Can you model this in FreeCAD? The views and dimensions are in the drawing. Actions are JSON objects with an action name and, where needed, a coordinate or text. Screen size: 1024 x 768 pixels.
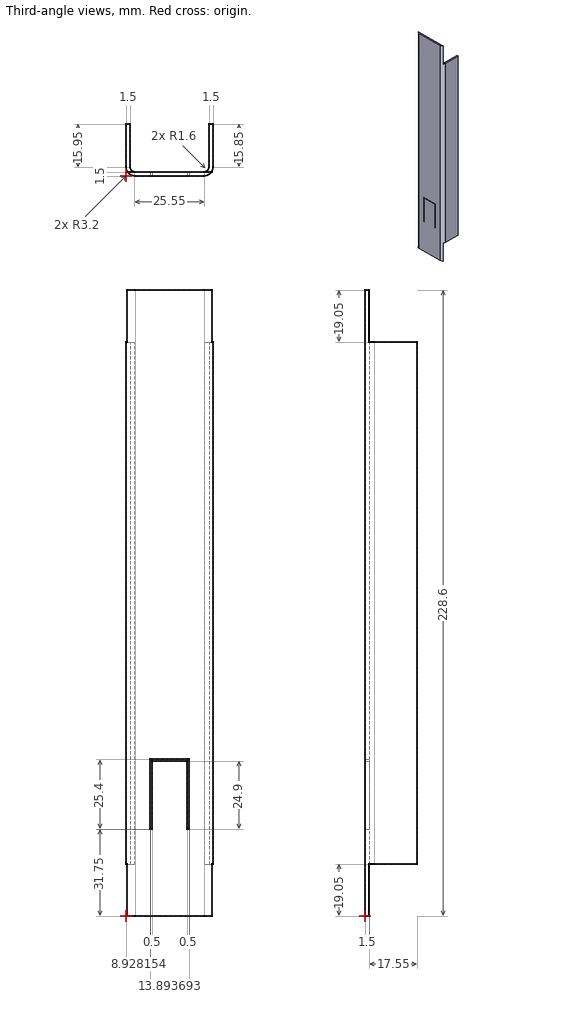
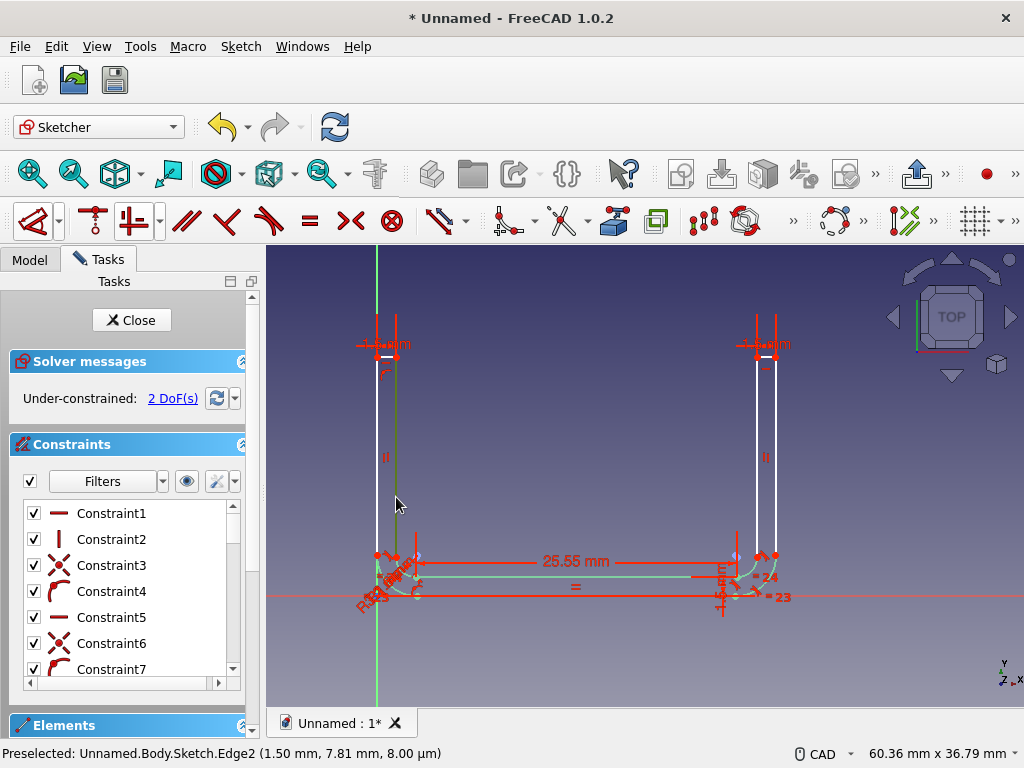
{"action": "left_click", "coordinate": [58, 222]}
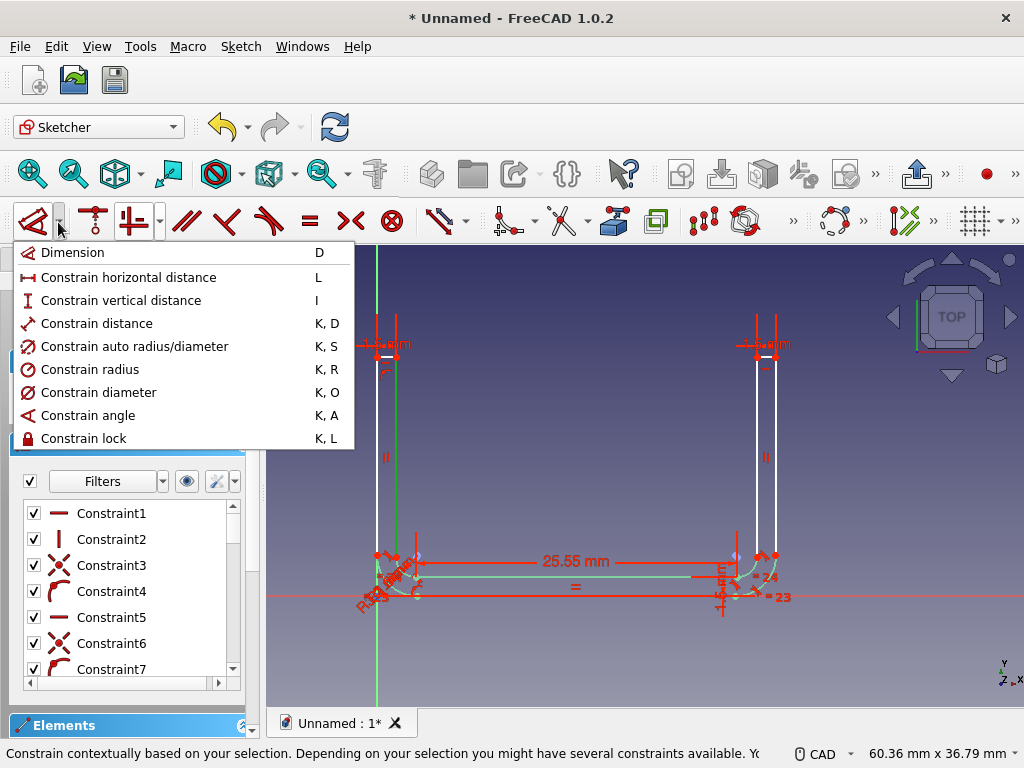
{"action": "left_click", "coordinate": [184, 300]}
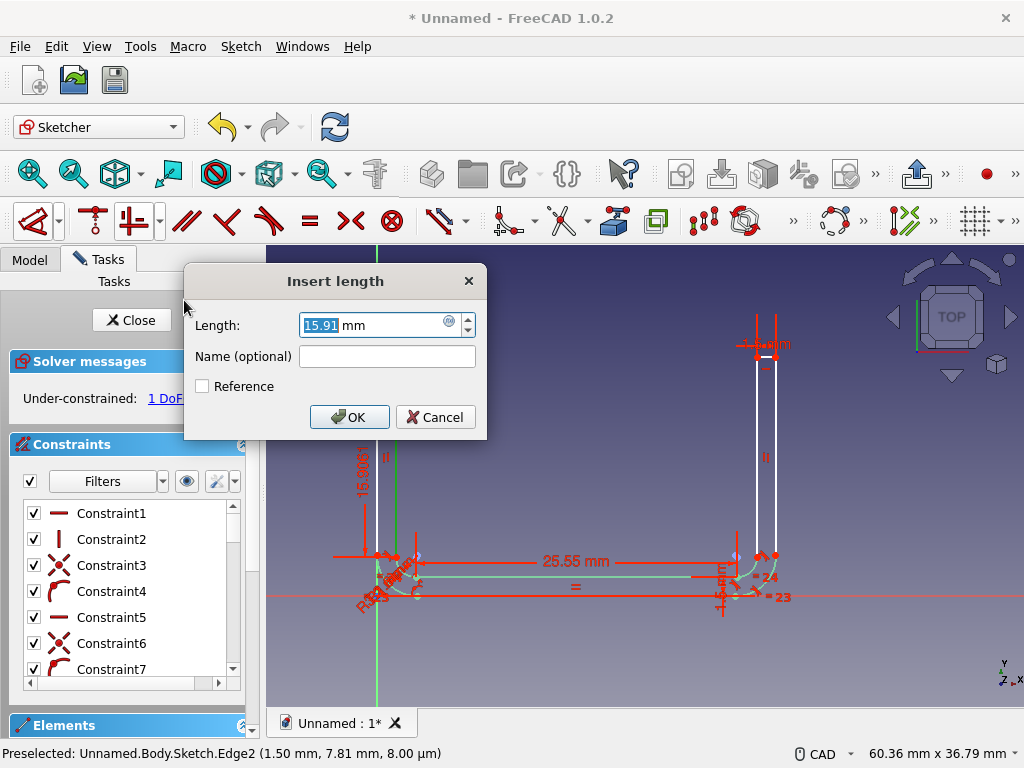
{"action": "type", "text": "15.95"}
{"action": "key", "text": "Return"}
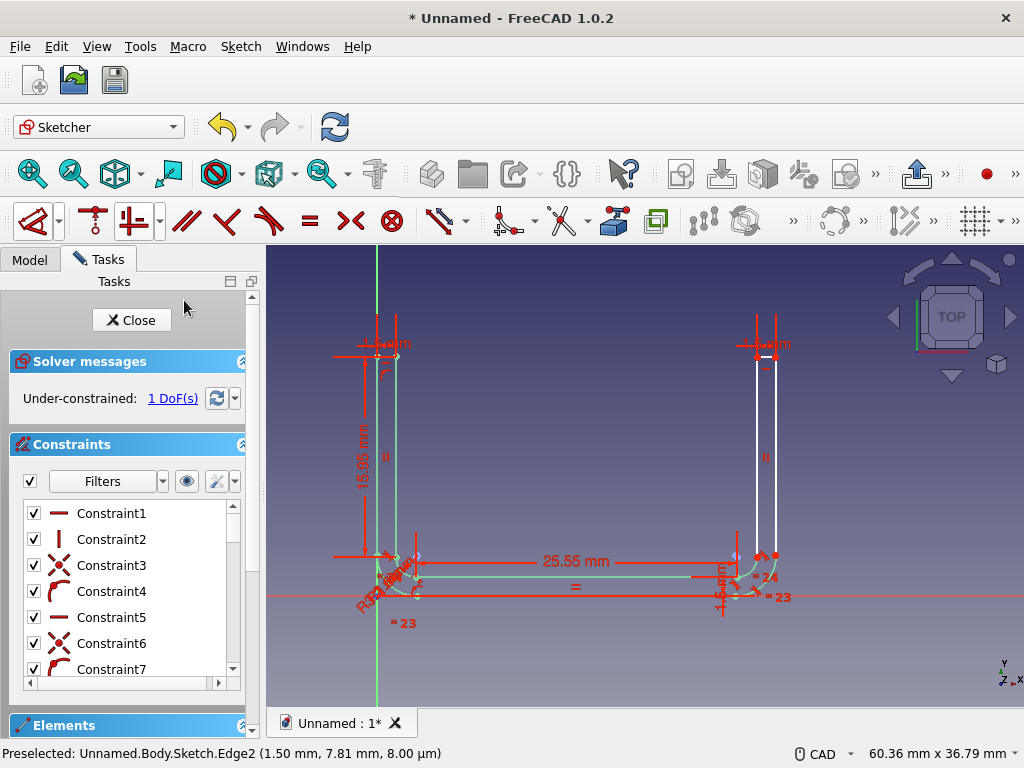
{"action": "left_click", "coordinate": [776, 496]}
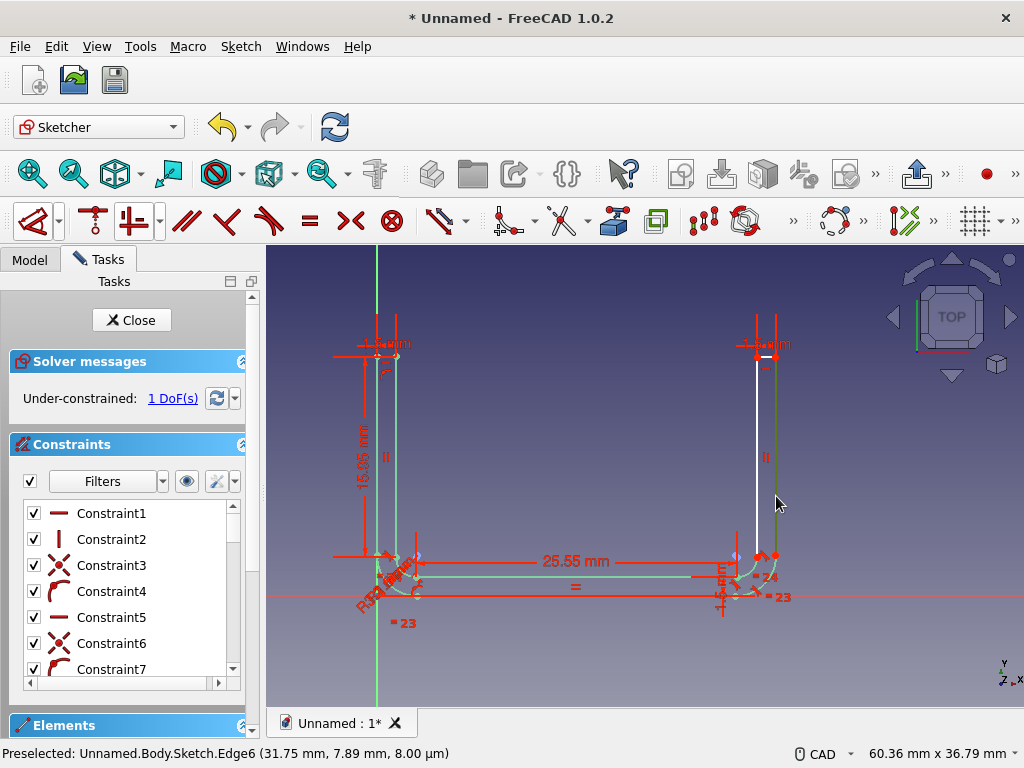
{"action": "left_click", "coordinate": [58, 222]}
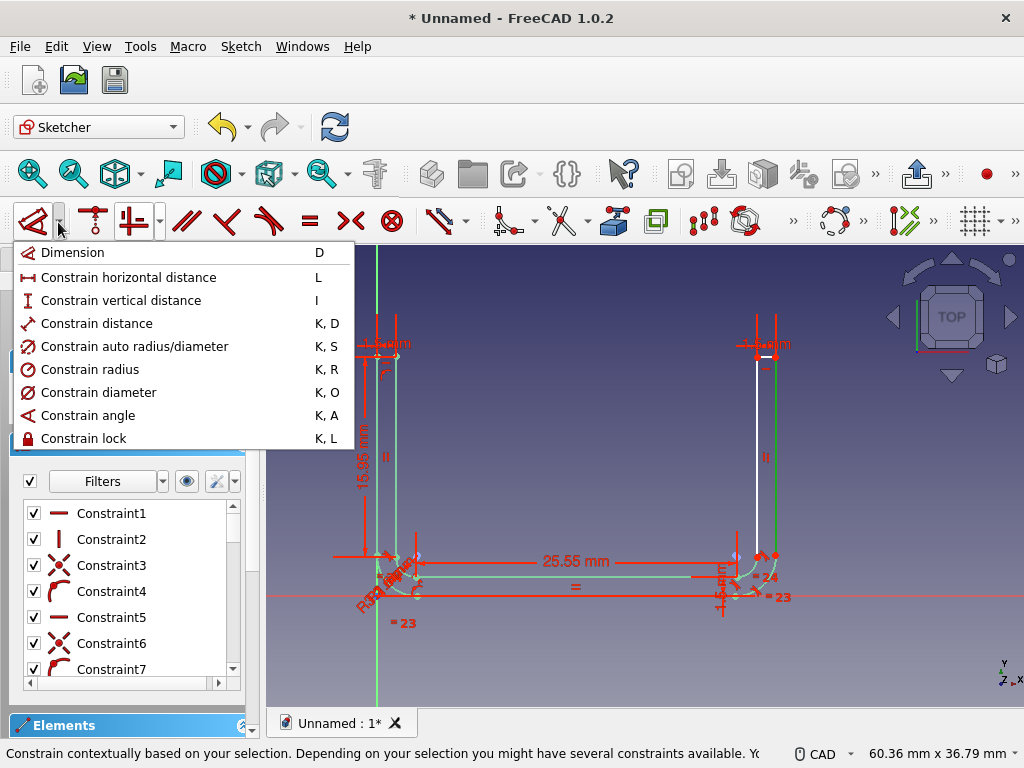
{"action": "left_click", "coordinate": [184, 300]}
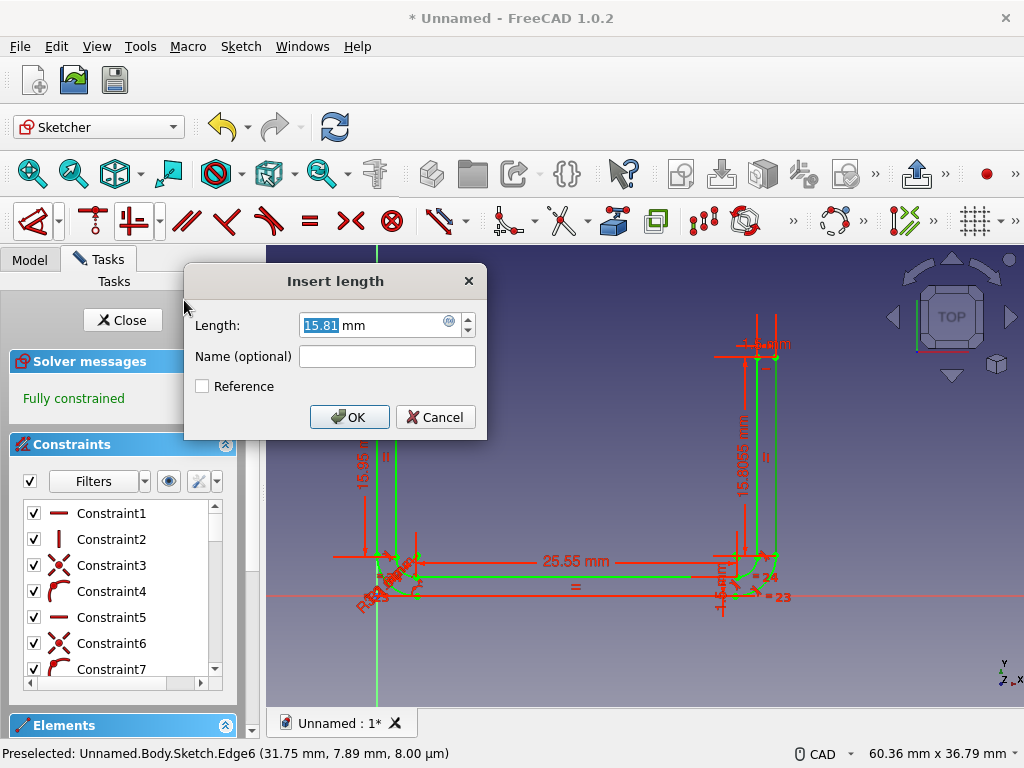
{"action": "type", "text": "15.85"}
{"action": "key", "text": "Return"}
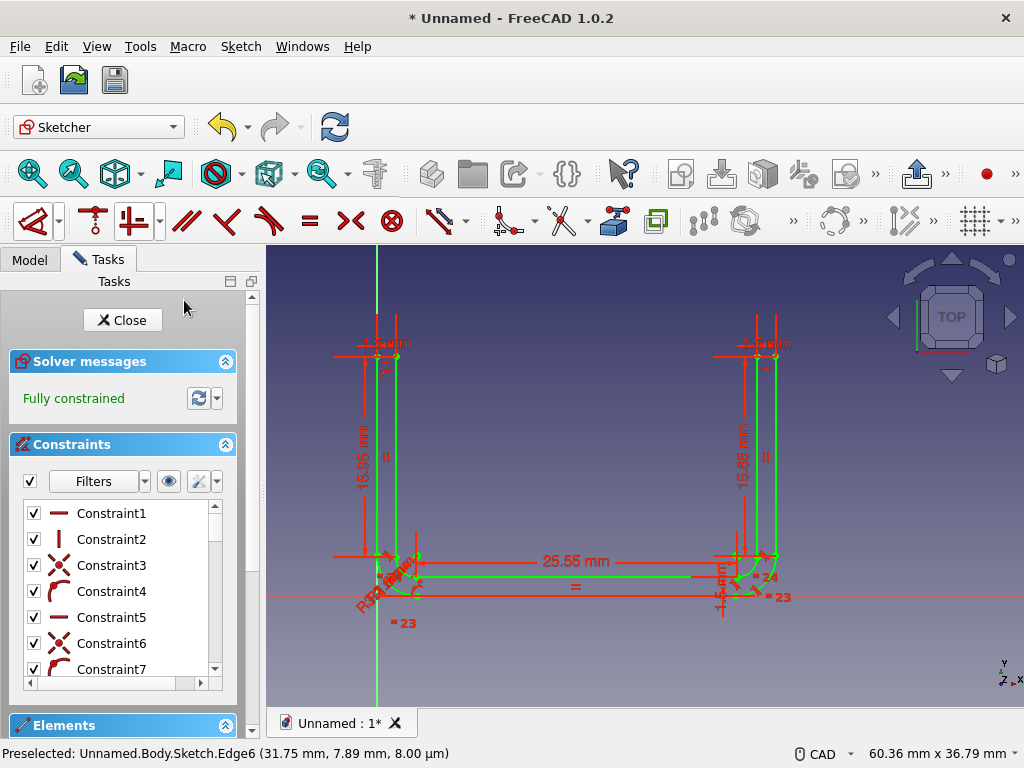
{"action": "left_click", "coordinate": [123, 320]}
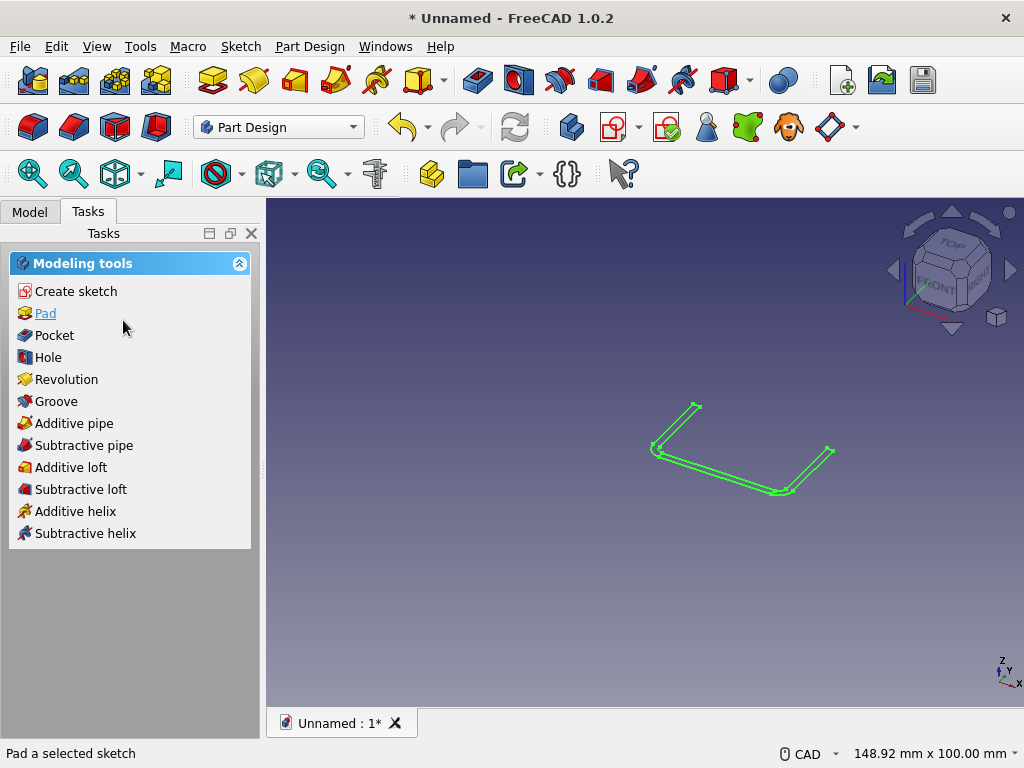
{"action": "left_click", "coordinate": [213, 80]}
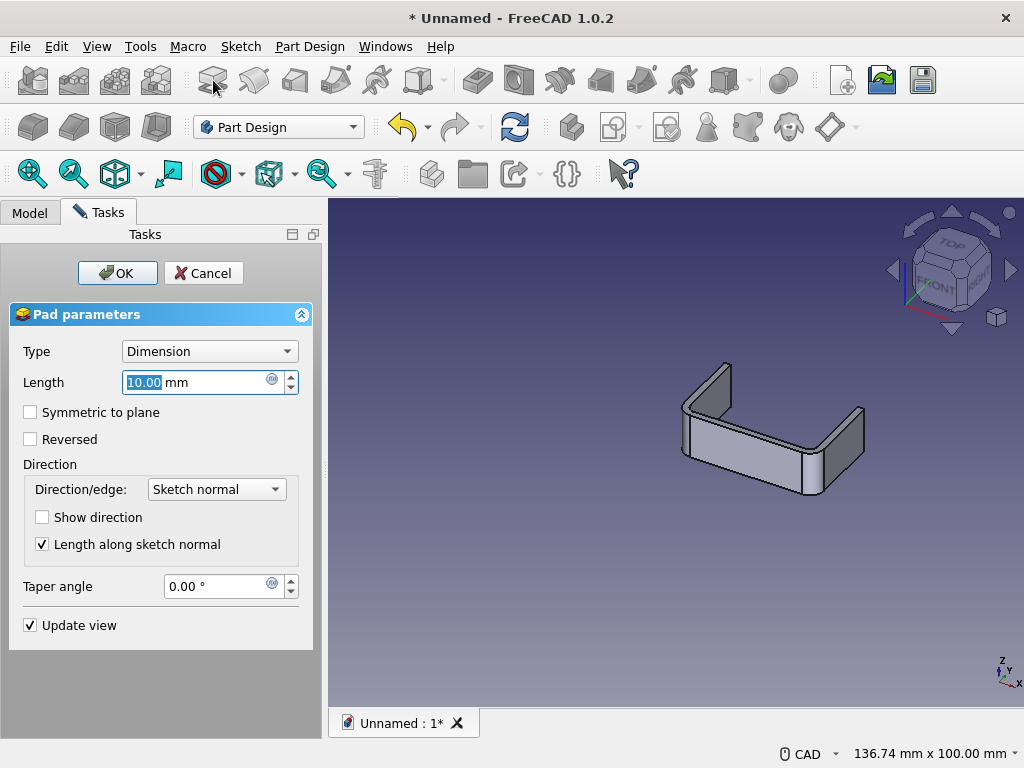
{"action": "type", "text": "228.6"}
{"action": "key", "text": "Tab"}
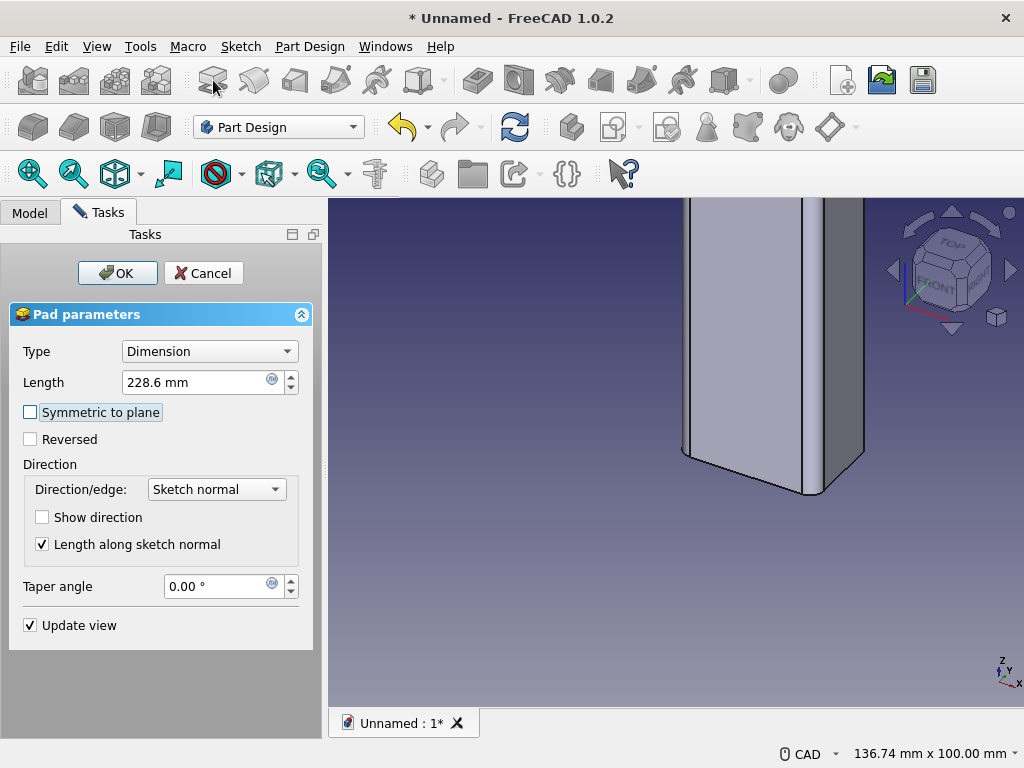
{"action": "left_click", "coordinate": [118, 273]}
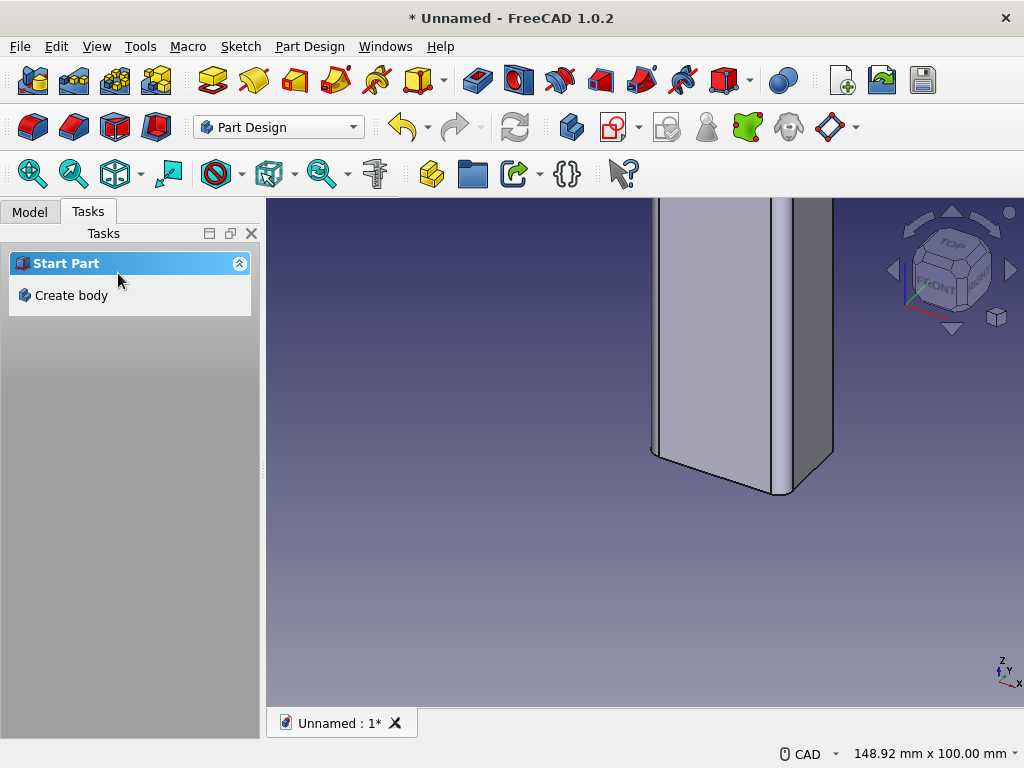
{"action": "left_click", "coordinate": [33, 174]}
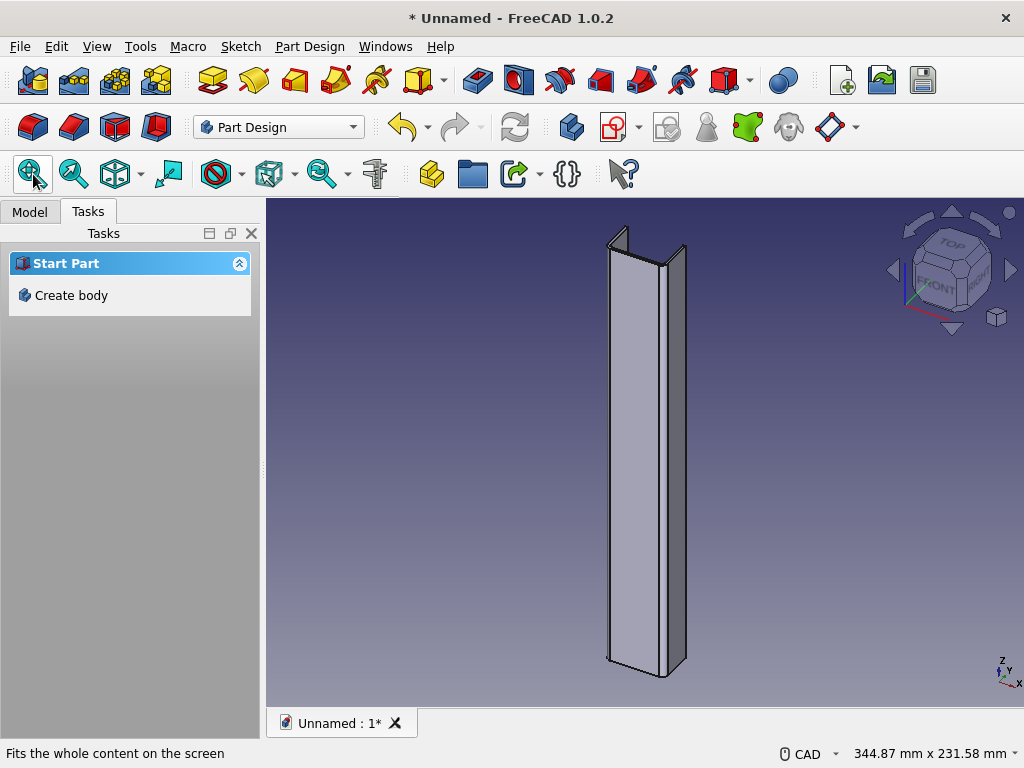
{"action": "left_click", "coordinate": [612, 128]}